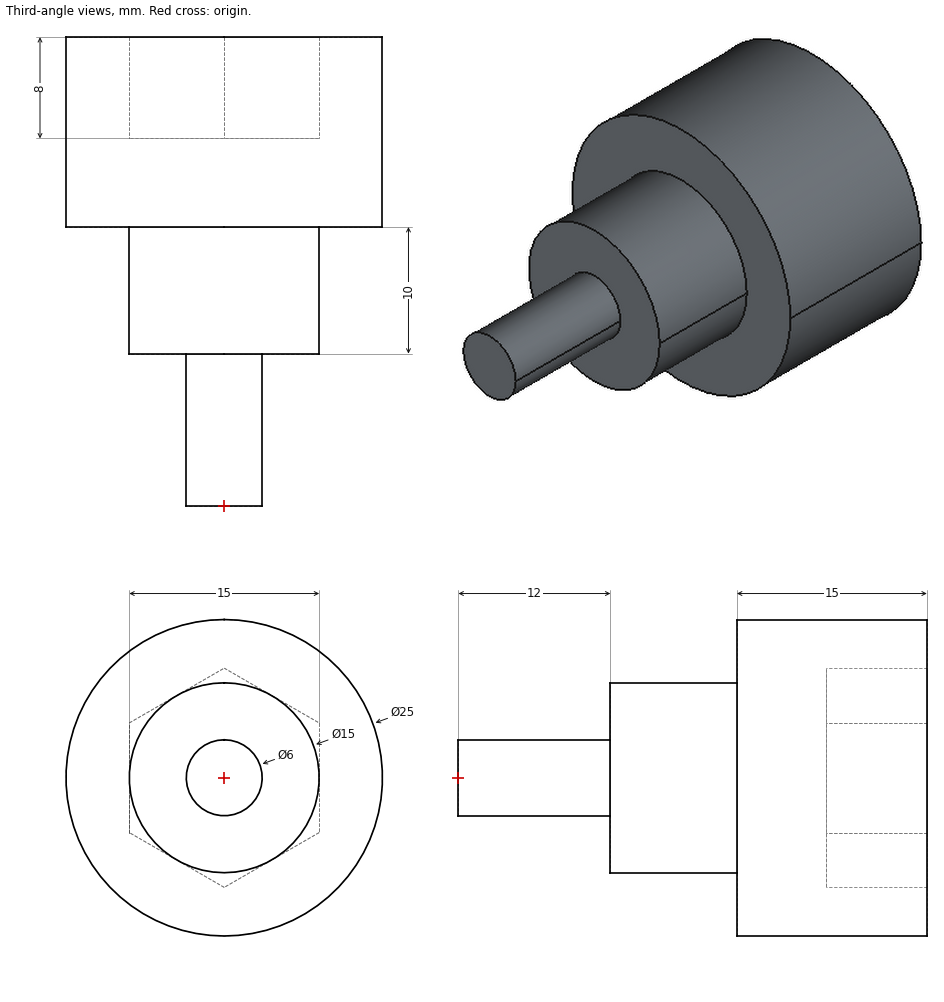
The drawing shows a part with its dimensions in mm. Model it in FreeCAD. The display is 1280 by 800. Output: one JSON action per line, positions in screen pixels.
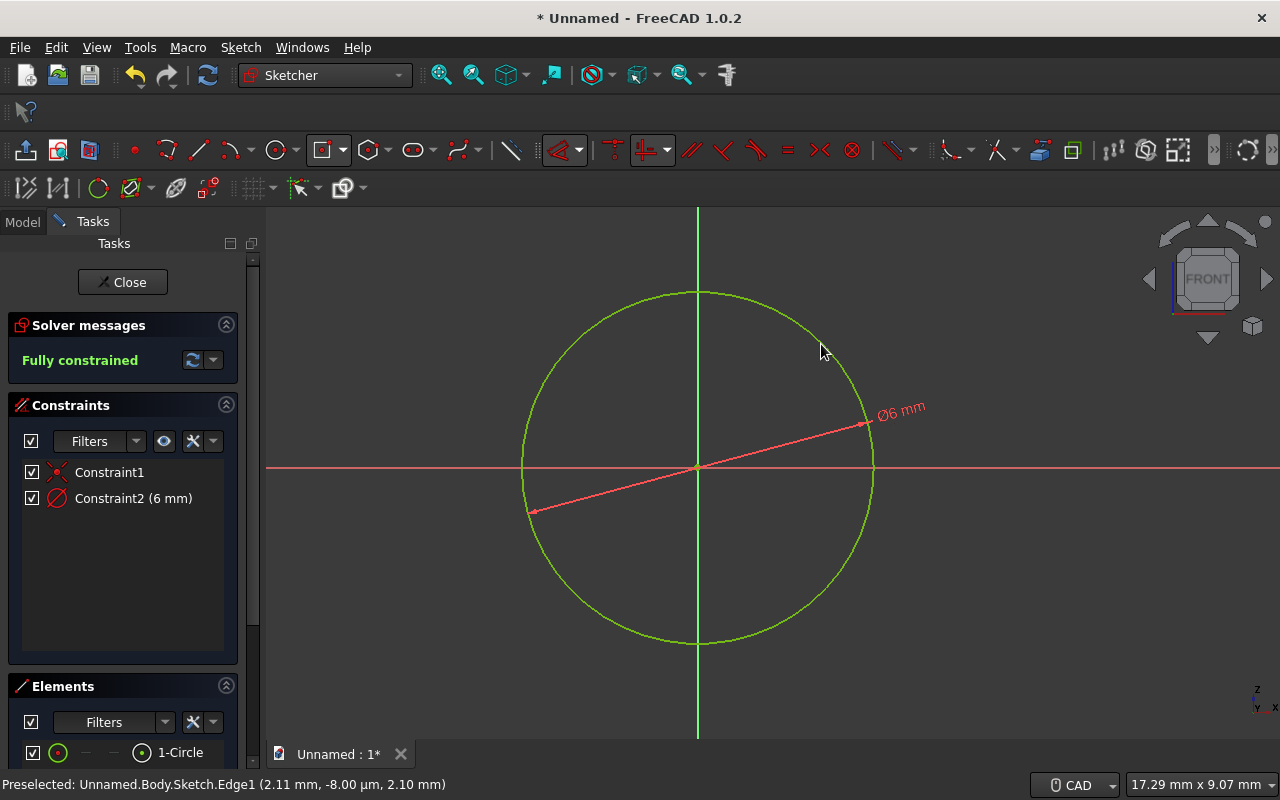
{"action": "left_click", "coordinate": [123, 282]}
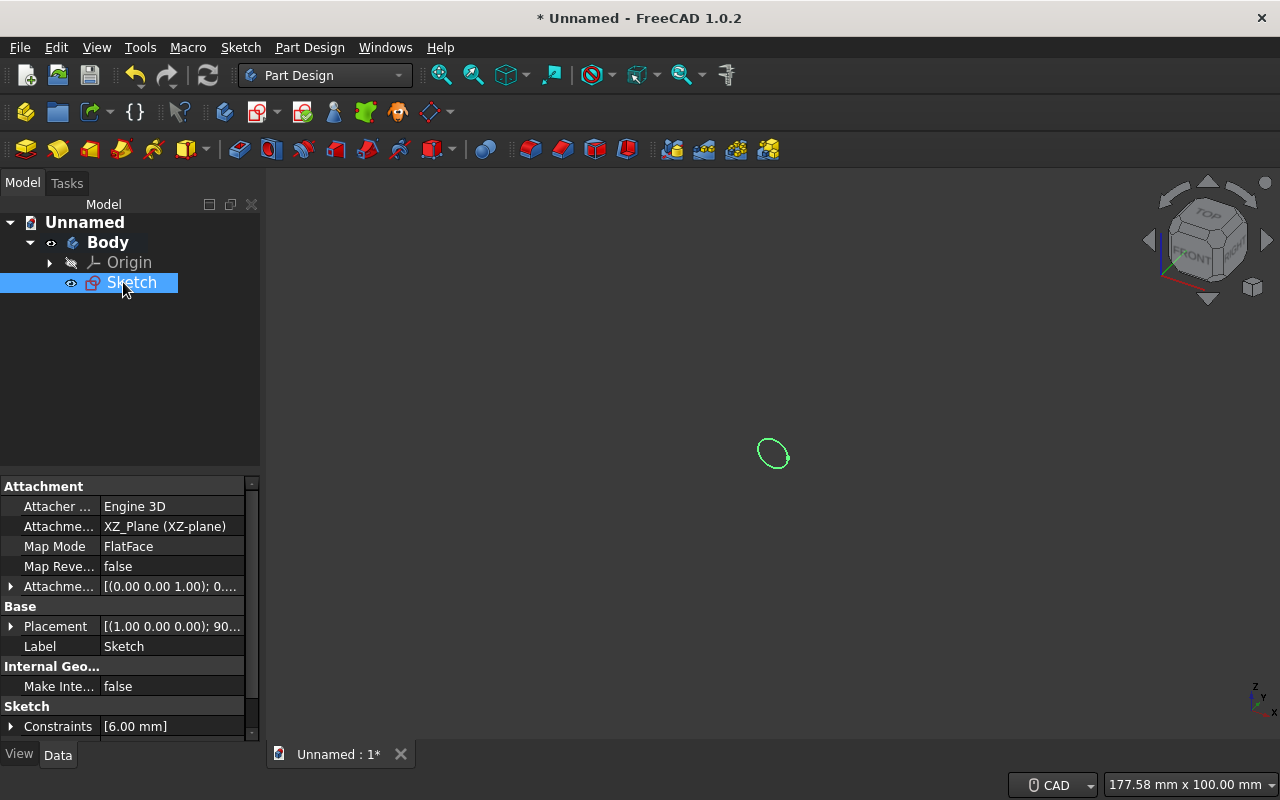
{"action": "left_click", "coordinate": [26, 150]}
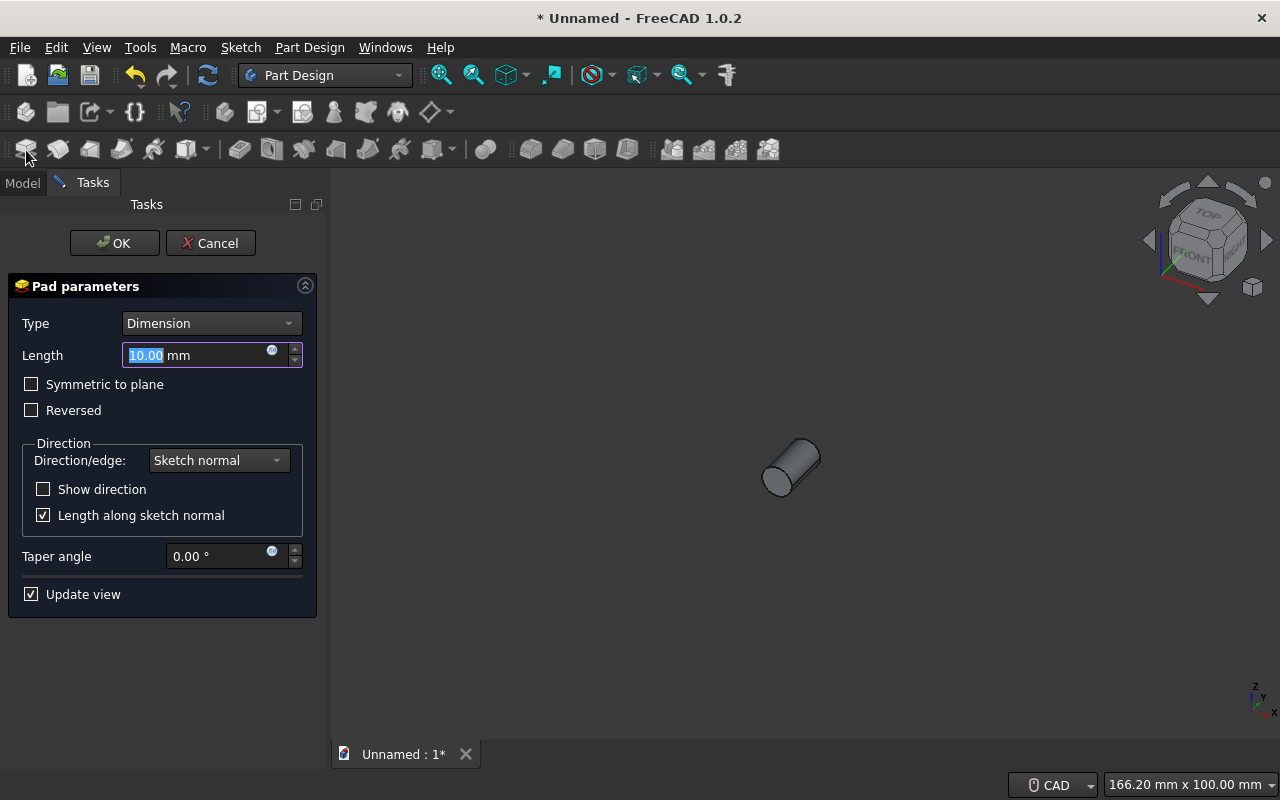
{"action": "type", "text": "12"}
{"action": "key", "text": "Tab"}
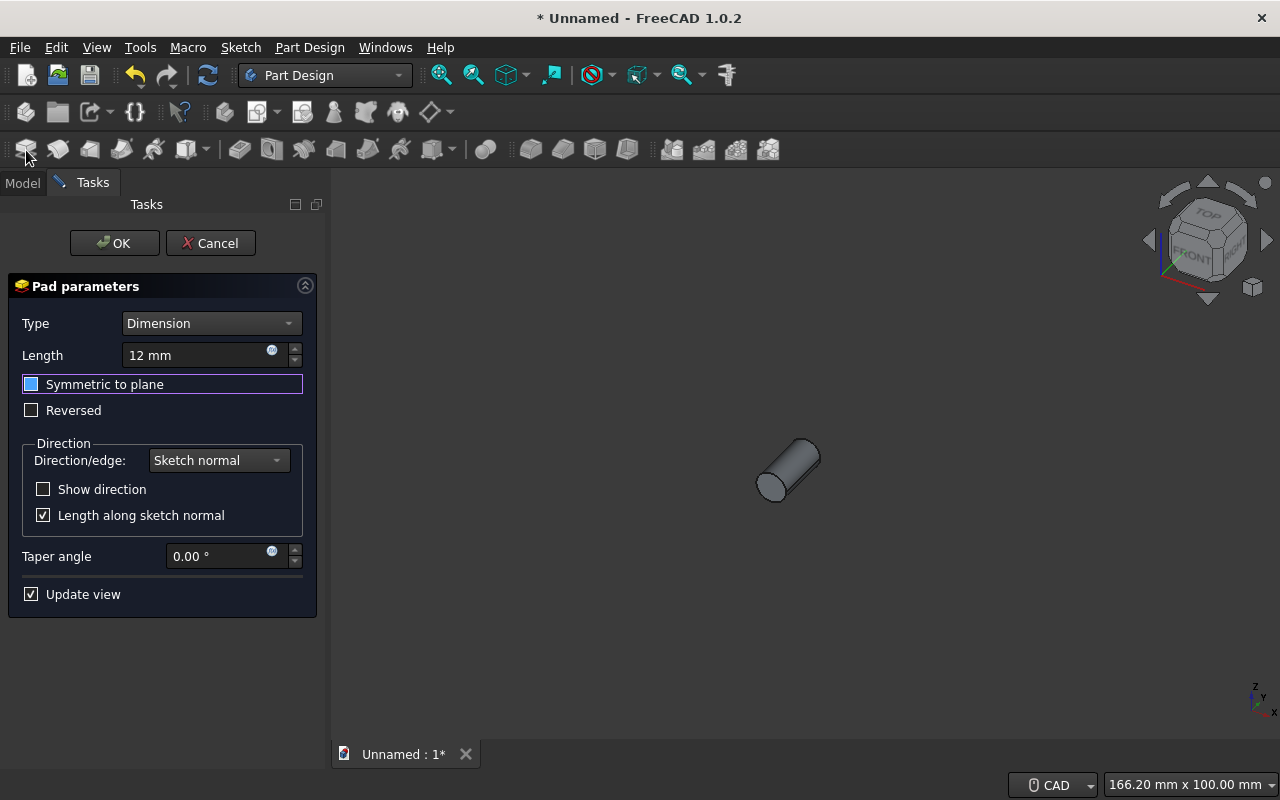
{"action": "left_click", "coordinate": [30, 410]}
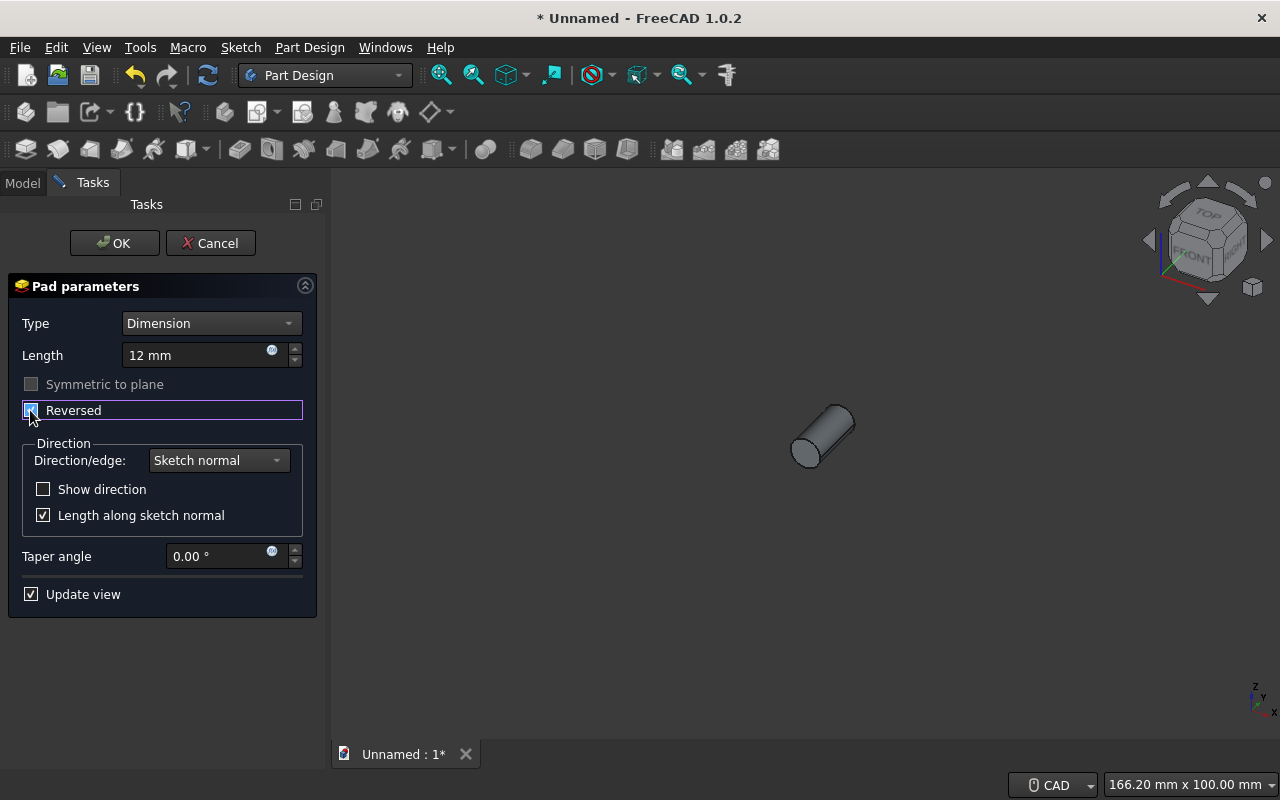
{"action": "left_click", "coordinate": [115, 243]}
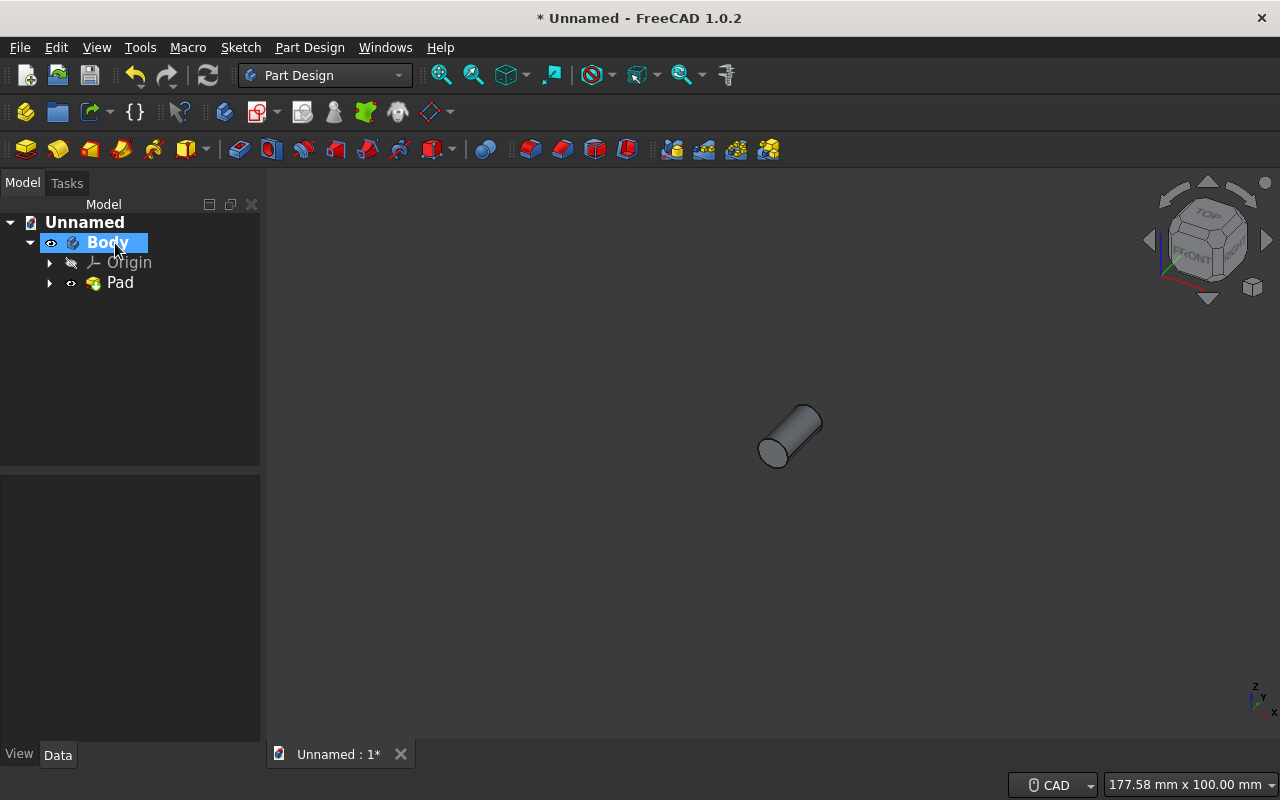
{"action": "left_click", "coordinate": [442, 76]}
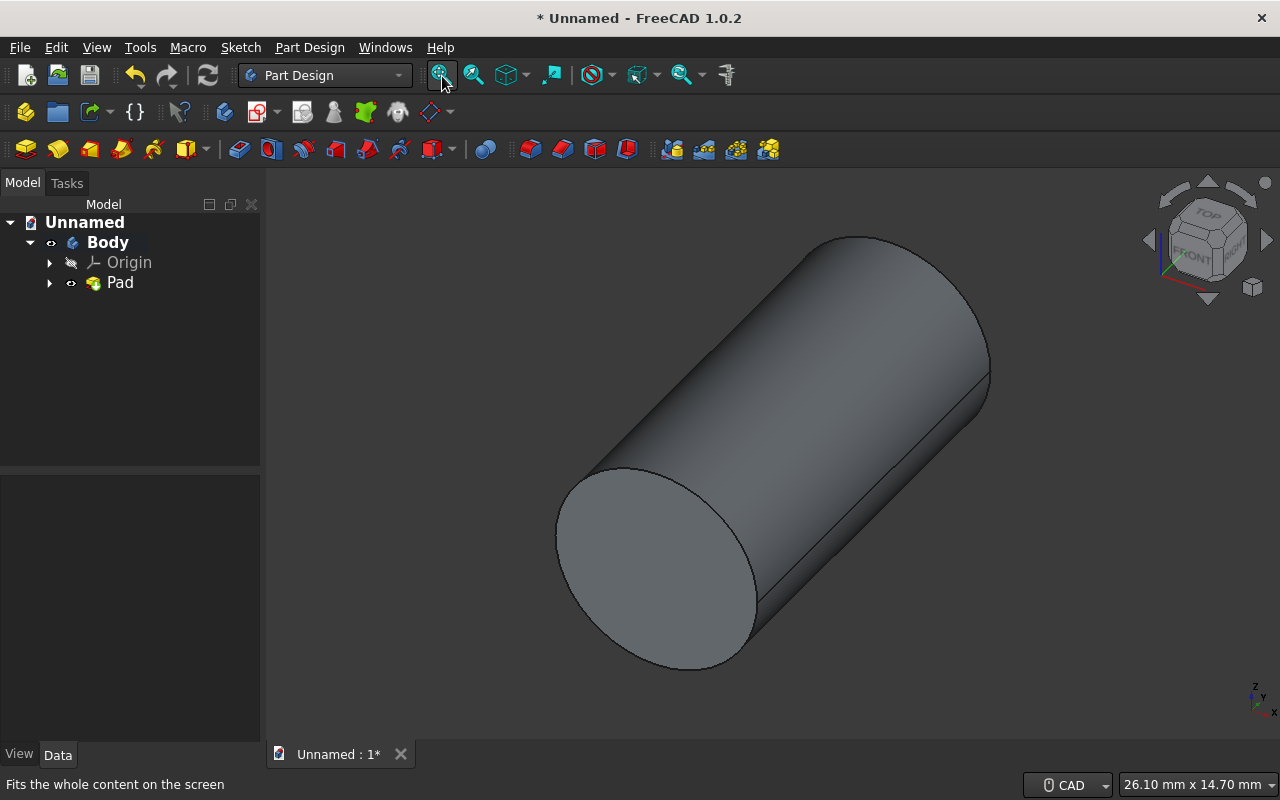
{"action": "key", "text": "4"}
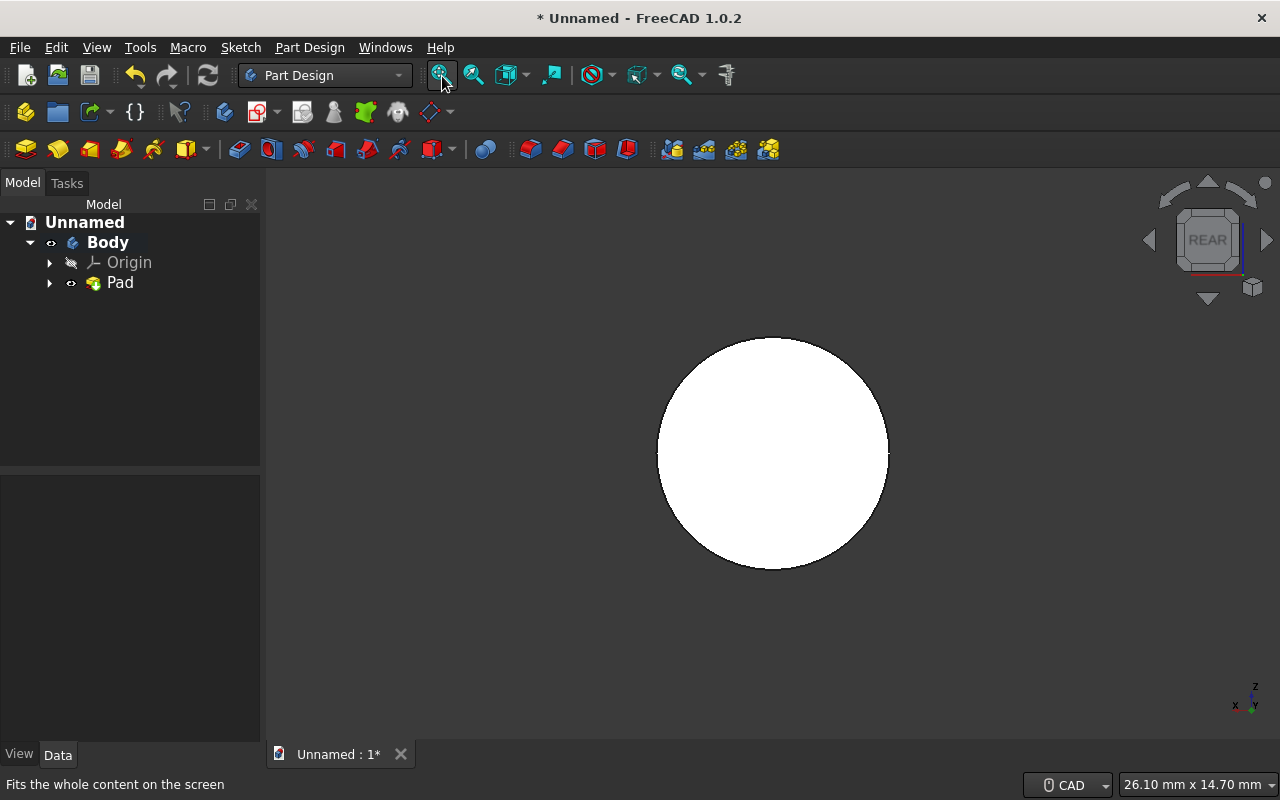
{"action": "key", "text": "v f"}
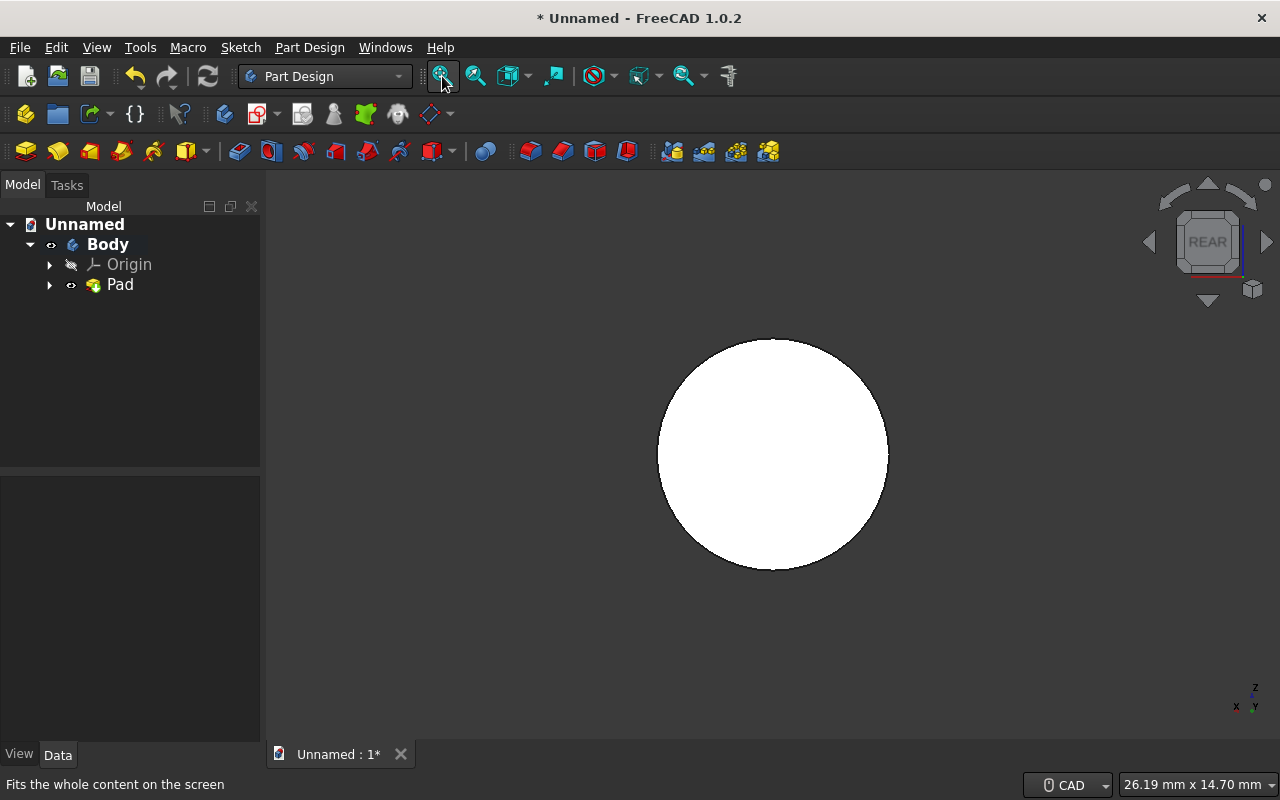
{"action": "left_click", "coordinate": [773, 454]}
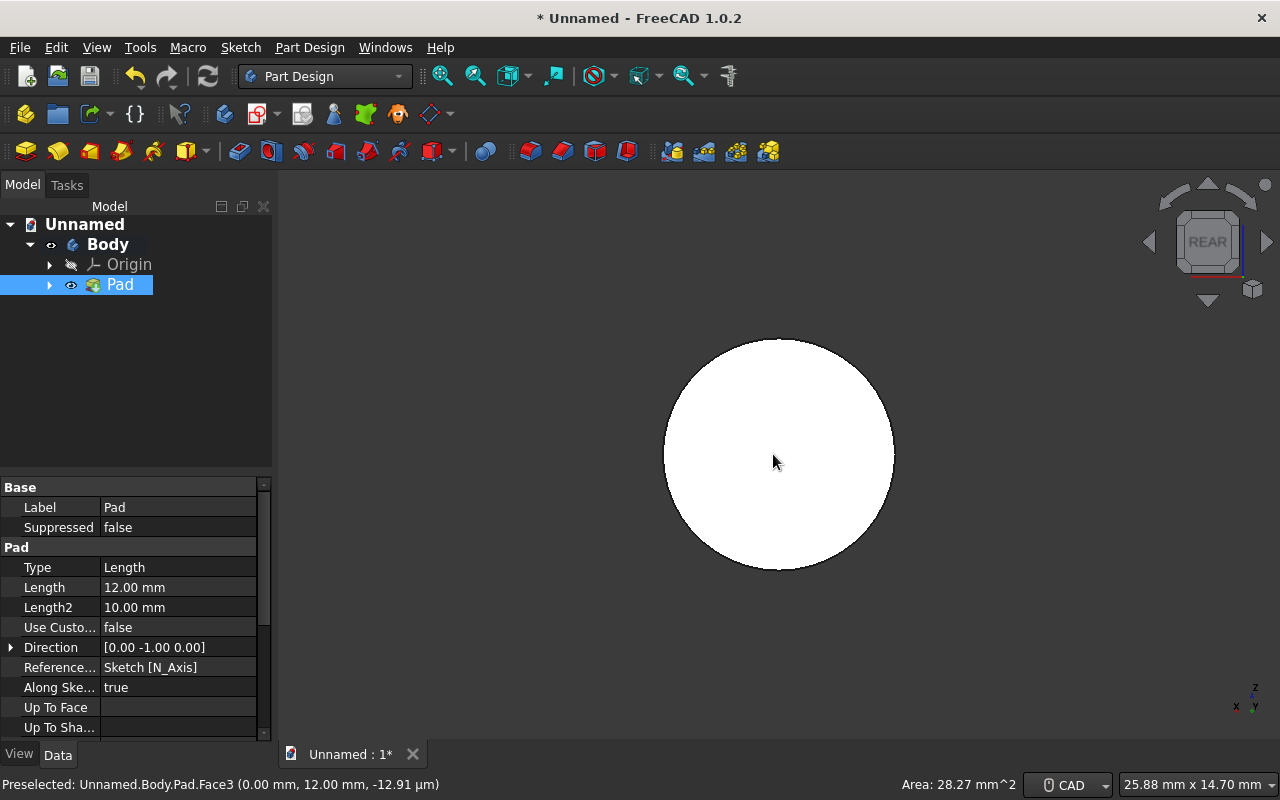
{"action": "left_click", "coordinate": [258, 114]}